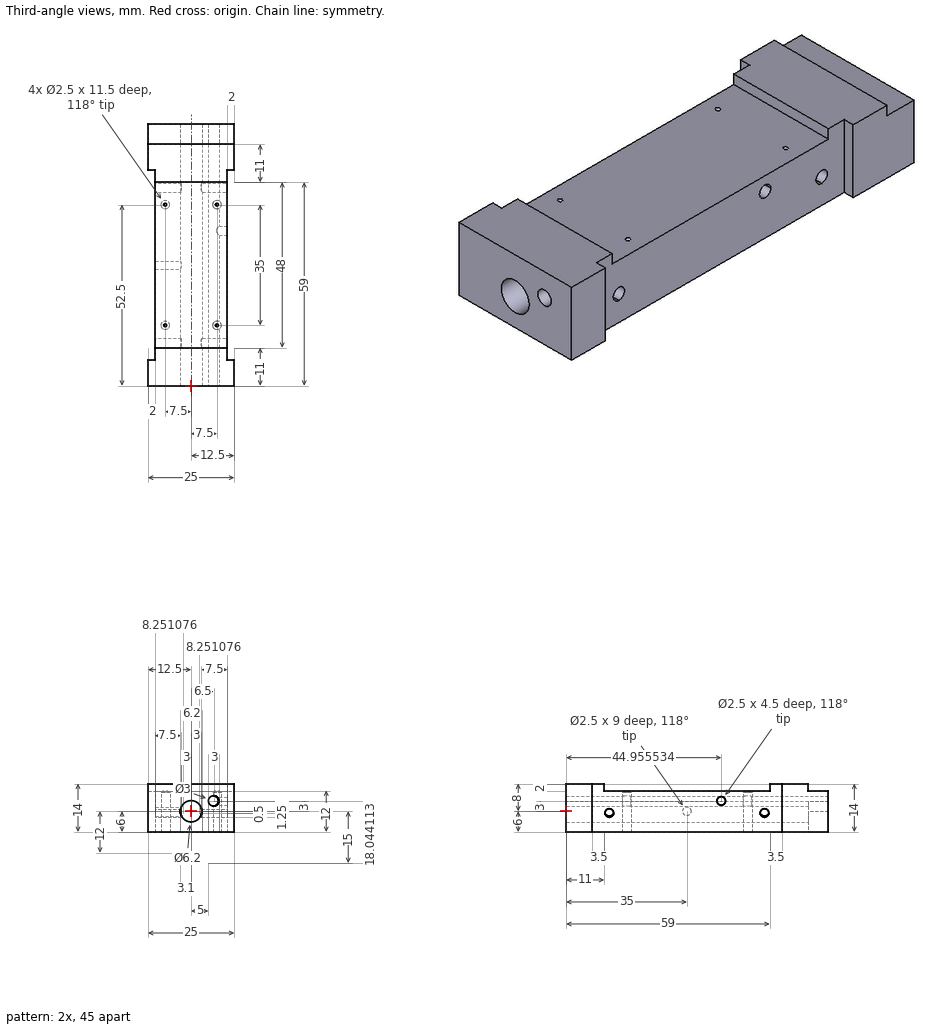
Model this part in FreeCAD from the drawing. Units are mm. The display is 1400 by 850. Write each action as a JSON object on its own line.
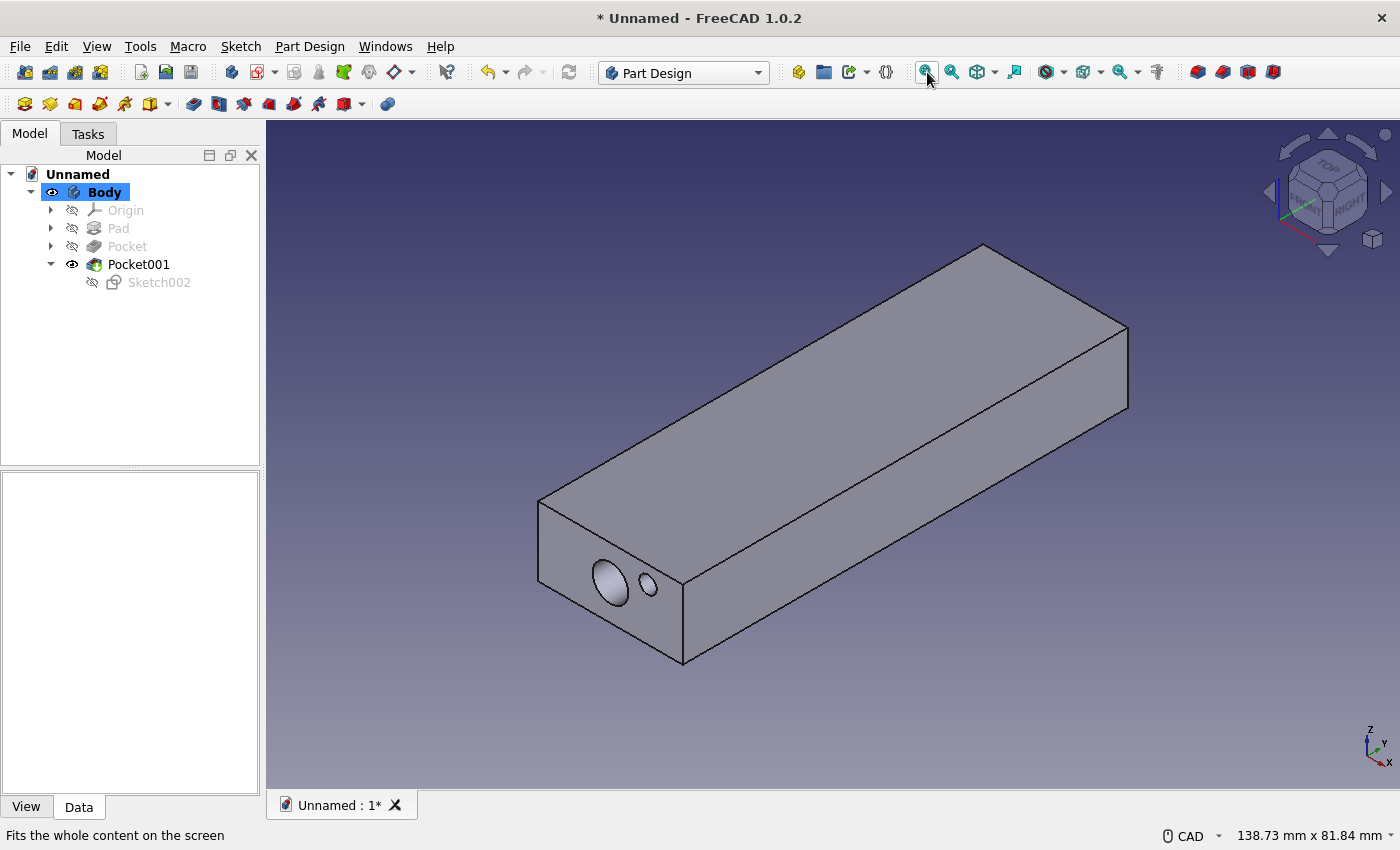
{"action": "left_click", "coordinate": [960, 340]}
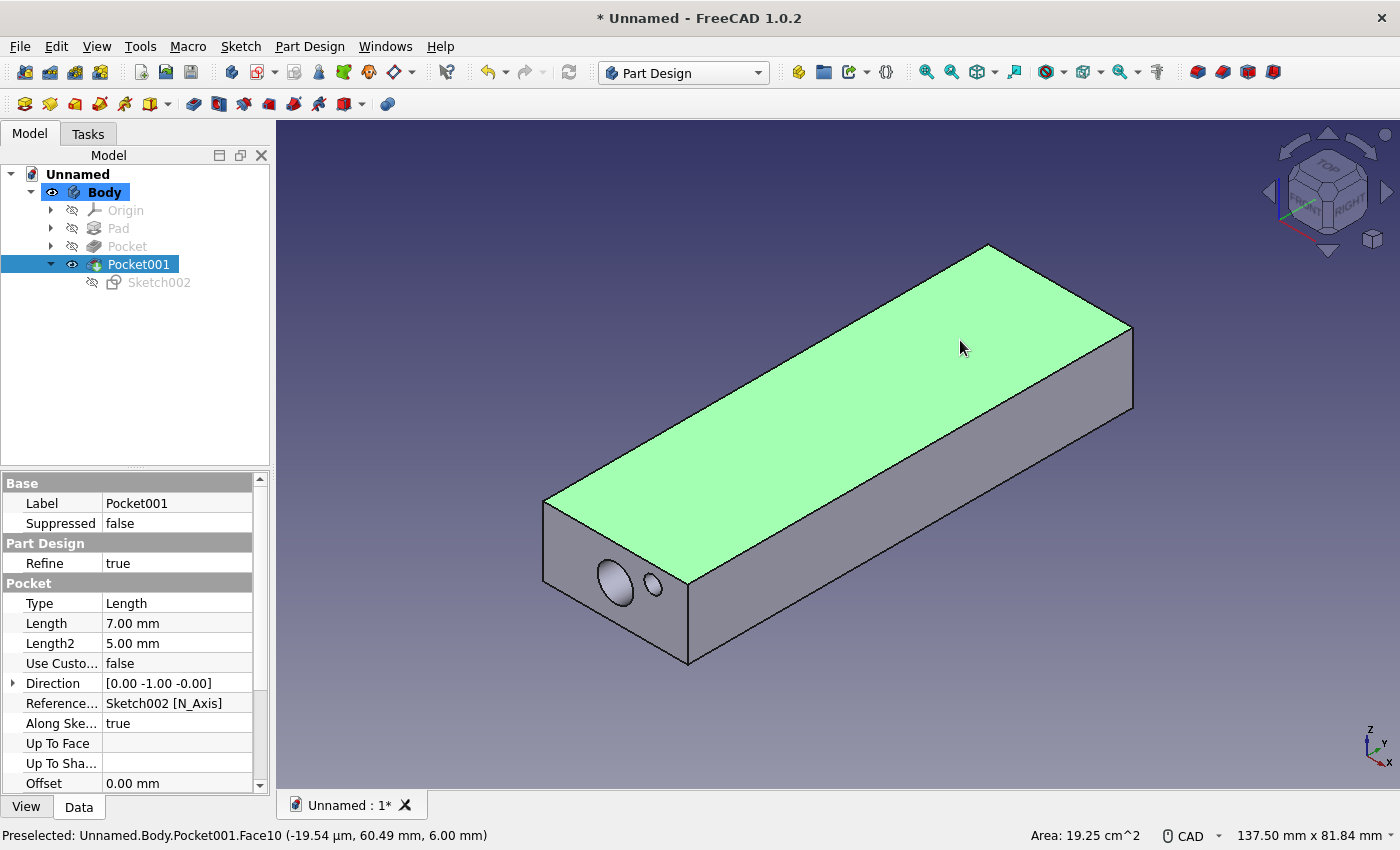
{"action": "left_click", "coordinate": [256, 72]}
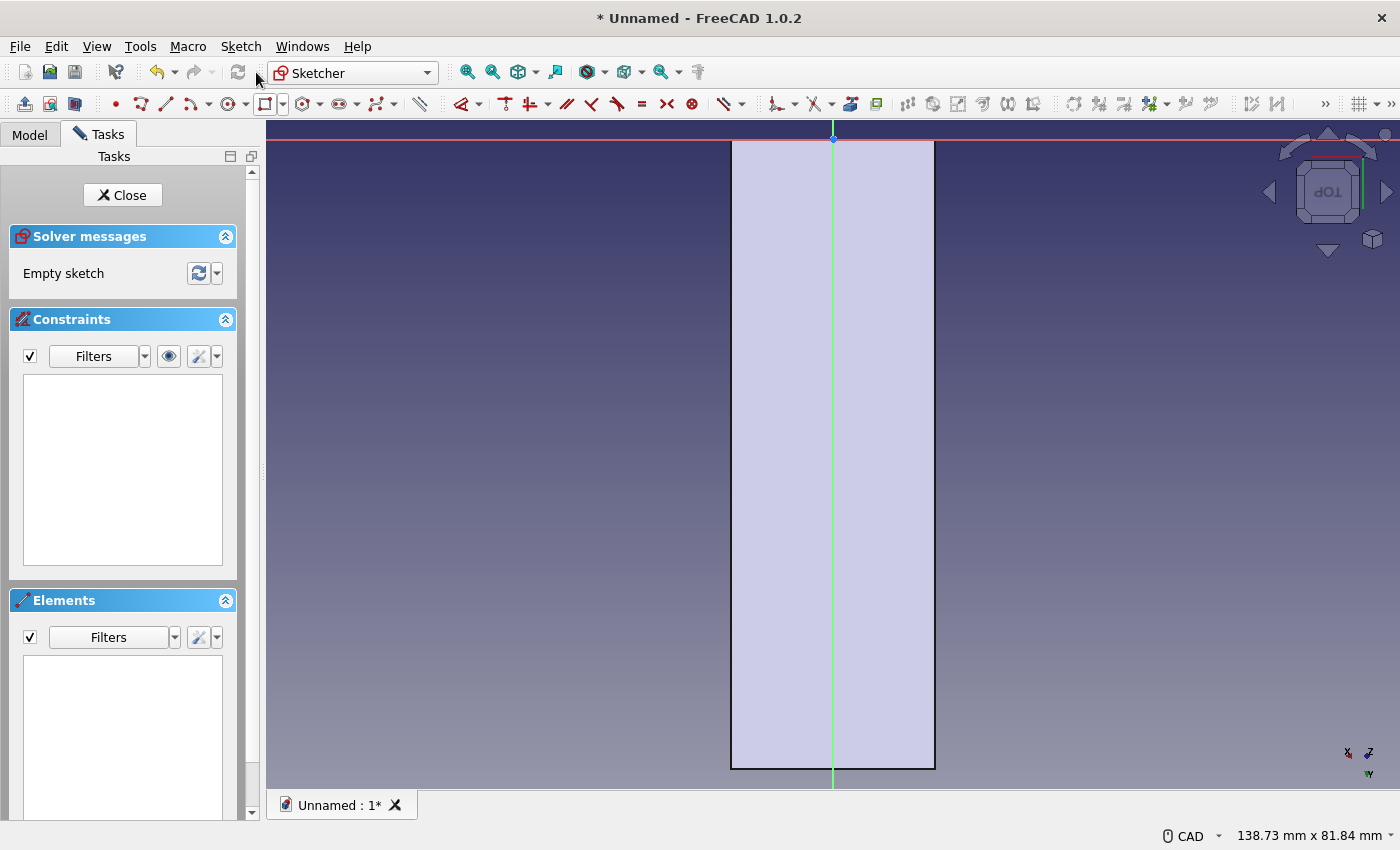
{"action": "scroll", "coordinate": [455, 584], "scroll_direction": "down", "scroll_amount": 1}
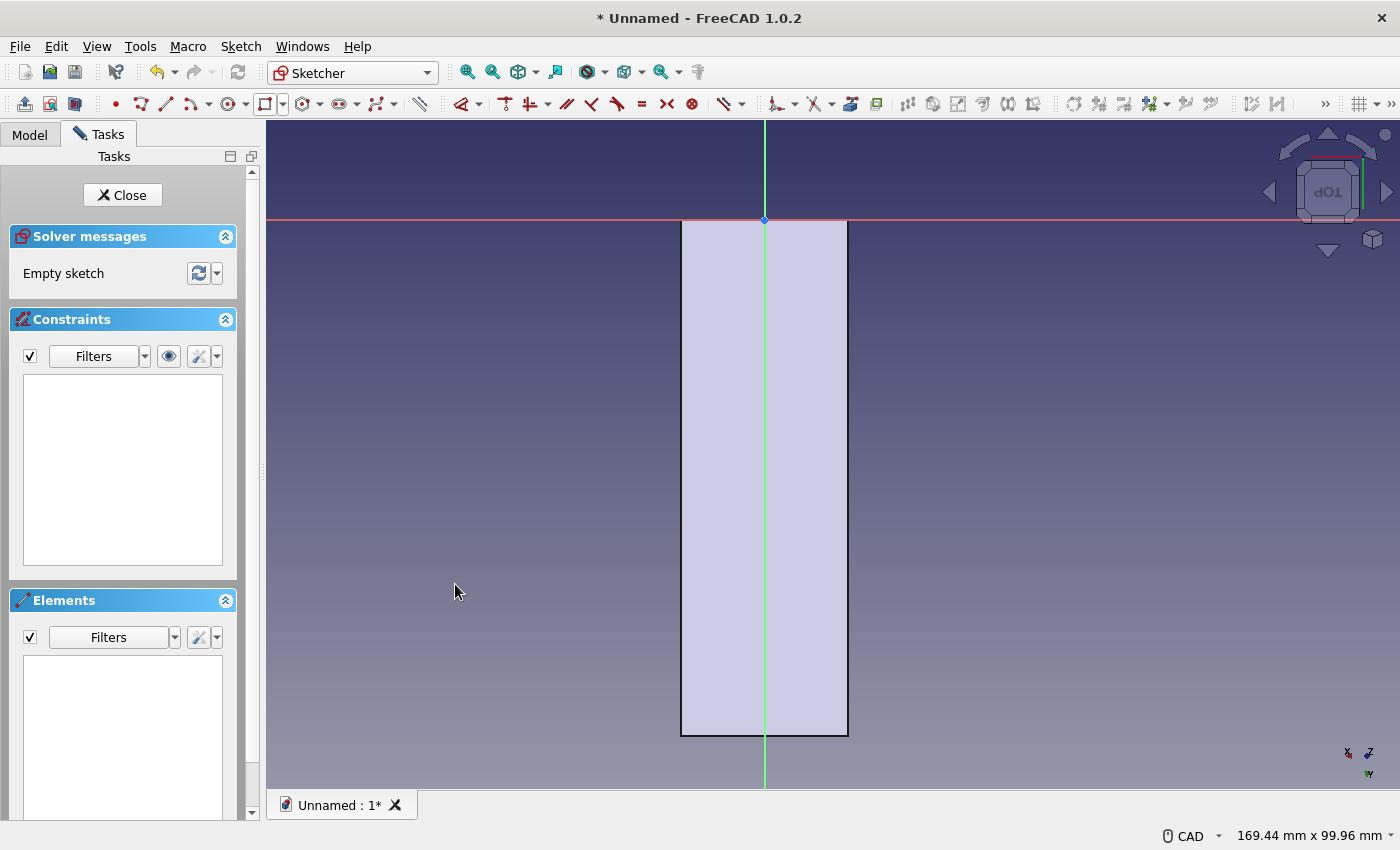
{"action": "left_click", "coordinate": [264, 104]}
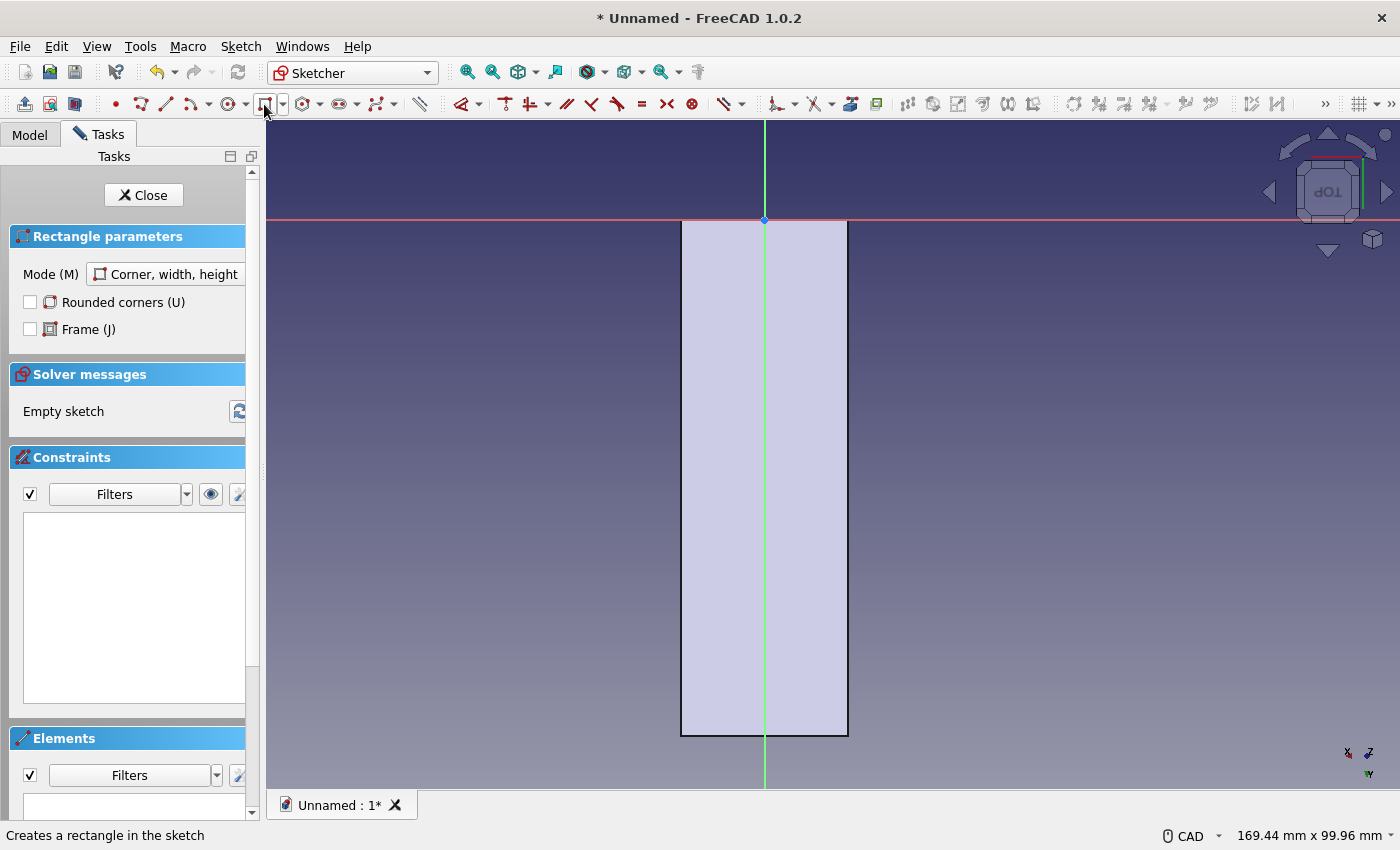
{"action": "left_click", "coordinate": [681, 220]}
{"action": "left_click", "coordinate": [848, 294]}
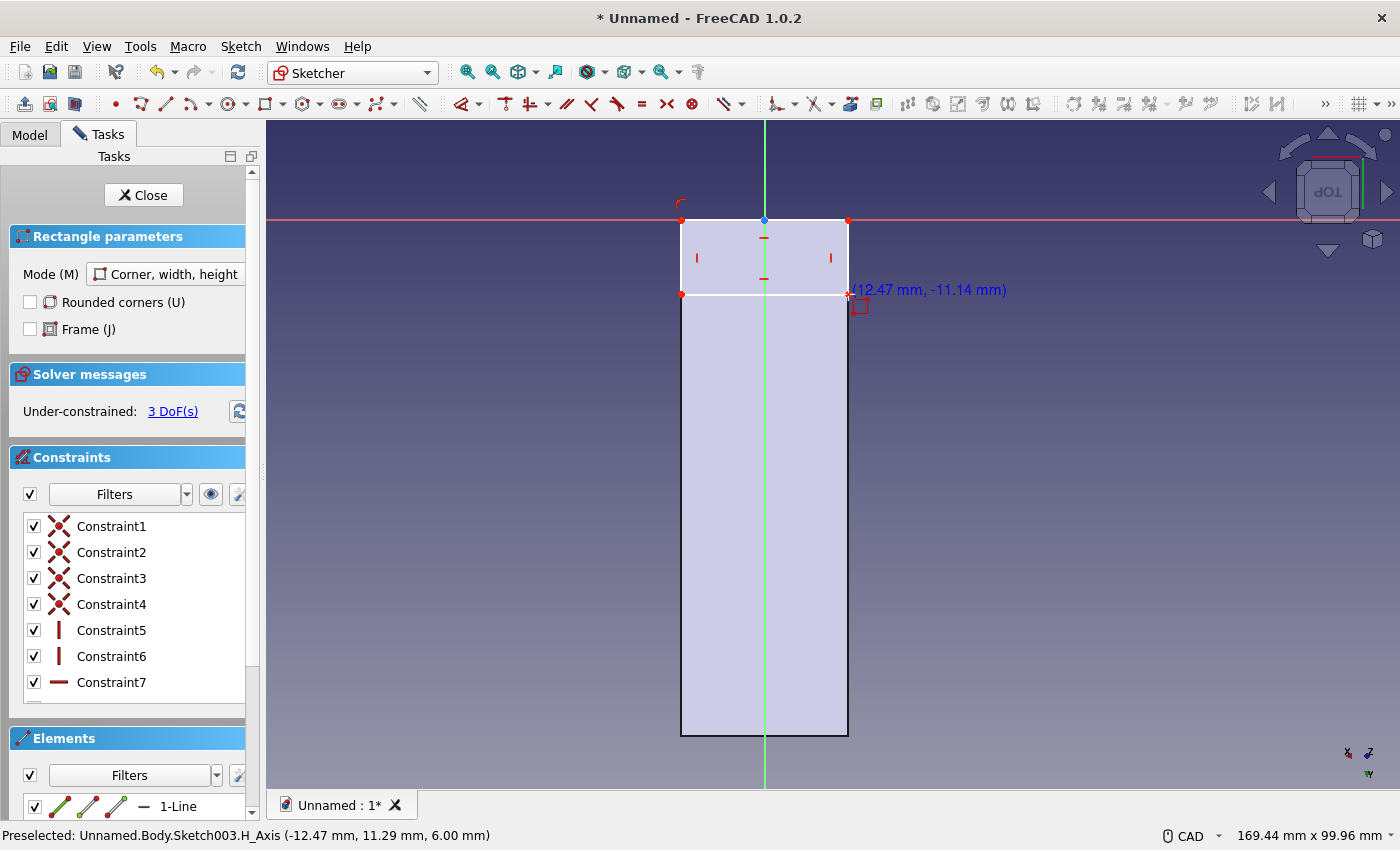
{"action": "left_click", "coordinate": [681, 615]}
{"action": "left_click", "coordinate": [848, 689]}
{"action": "key", "text": "Escape"}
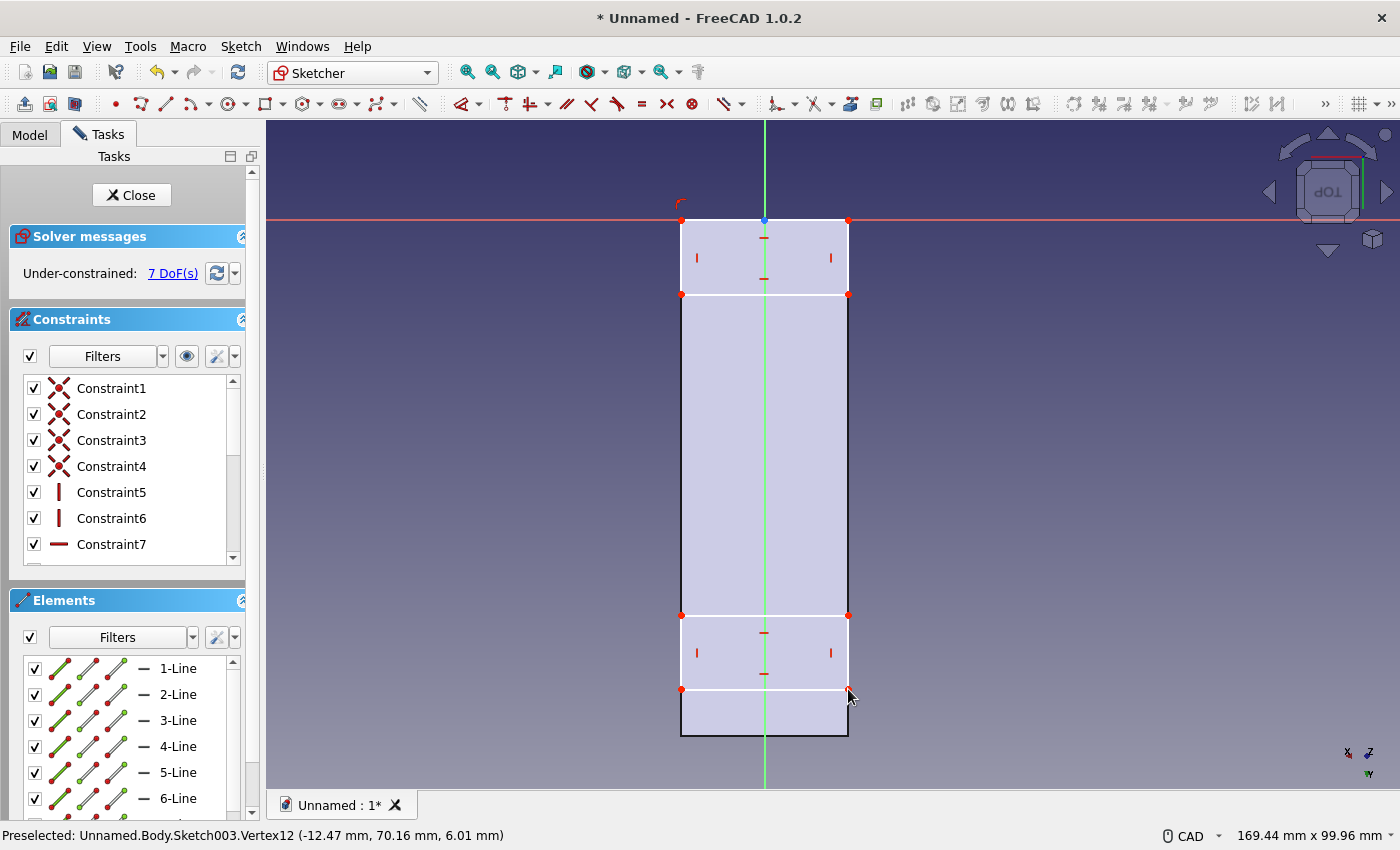
{"action": "left_click", "coordinate": [460, 104]}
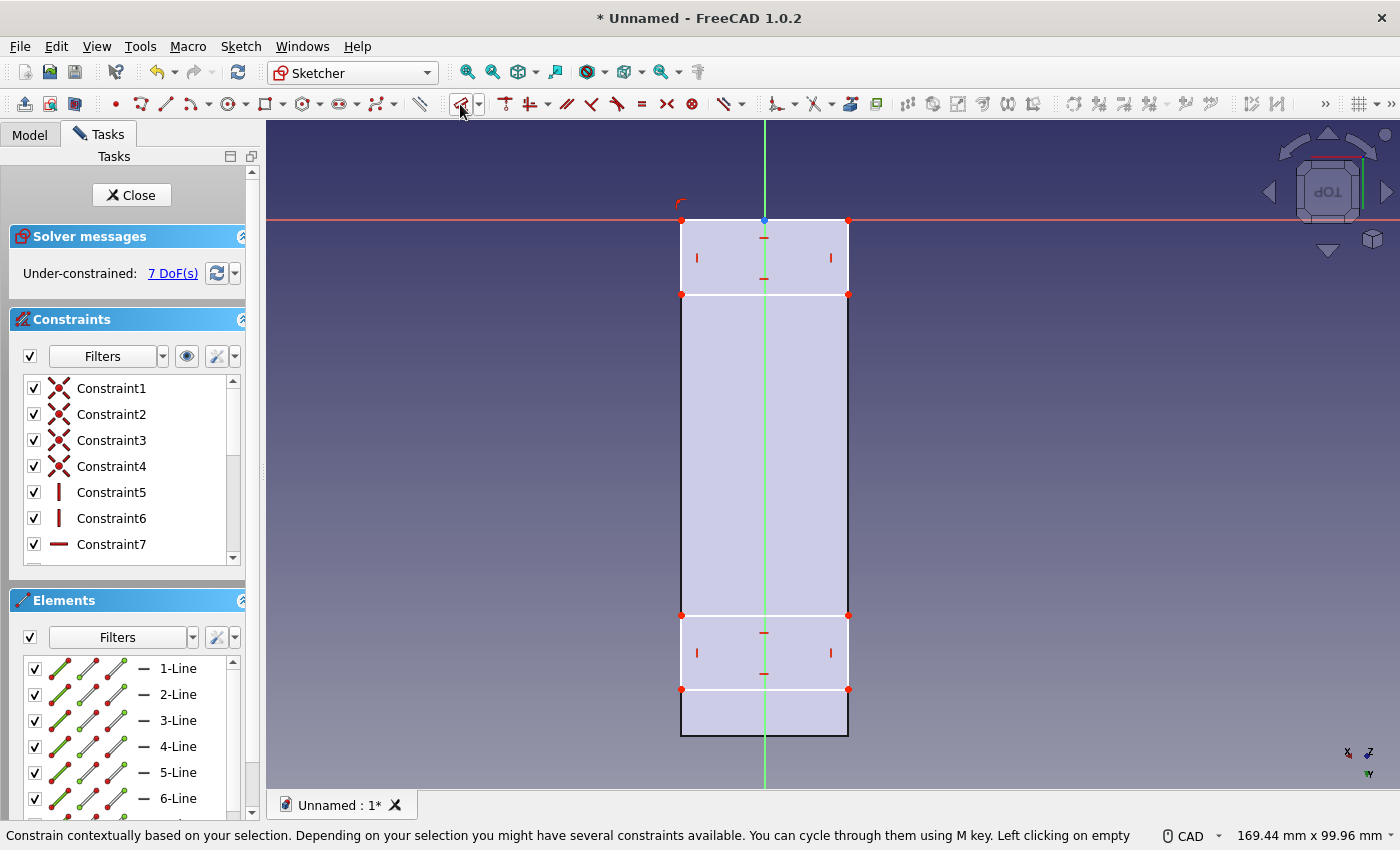
{"action": "left_click", "coordinate": [681, 243]}
{"action": "left_click", "coordinate": [647, 258]}